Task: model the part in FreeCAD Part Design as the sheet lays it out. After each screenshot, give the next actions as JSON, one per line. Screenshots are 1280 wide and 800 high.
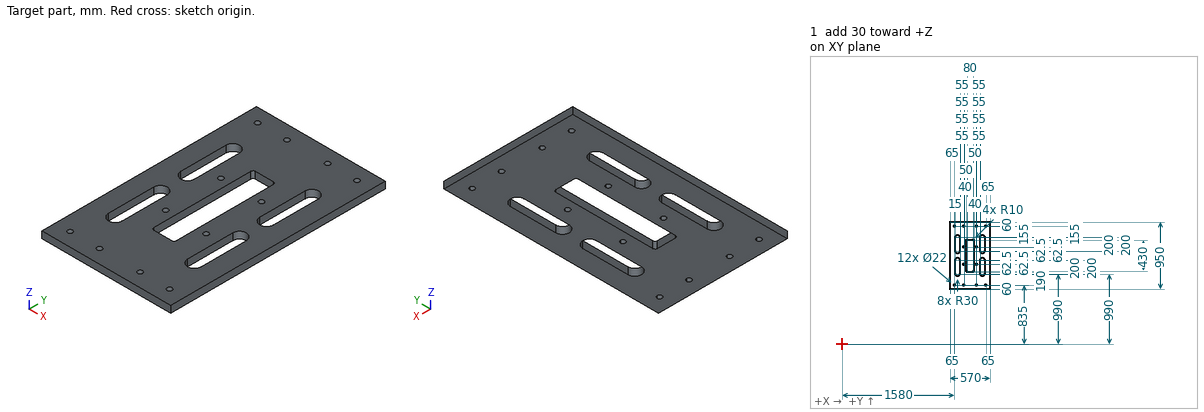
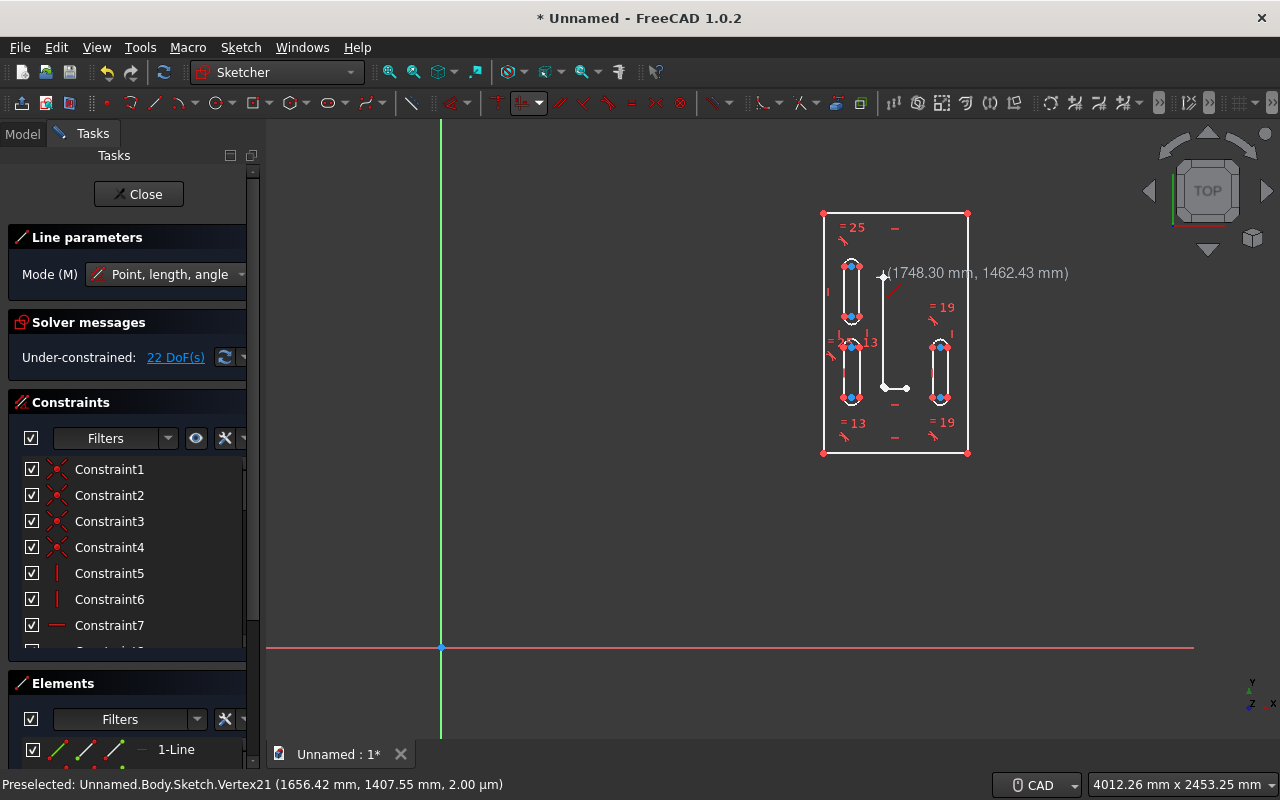
{"action": "scroll", "coordinate": [886, 275], "scroll_direction": "up", "scroll_amount": 8}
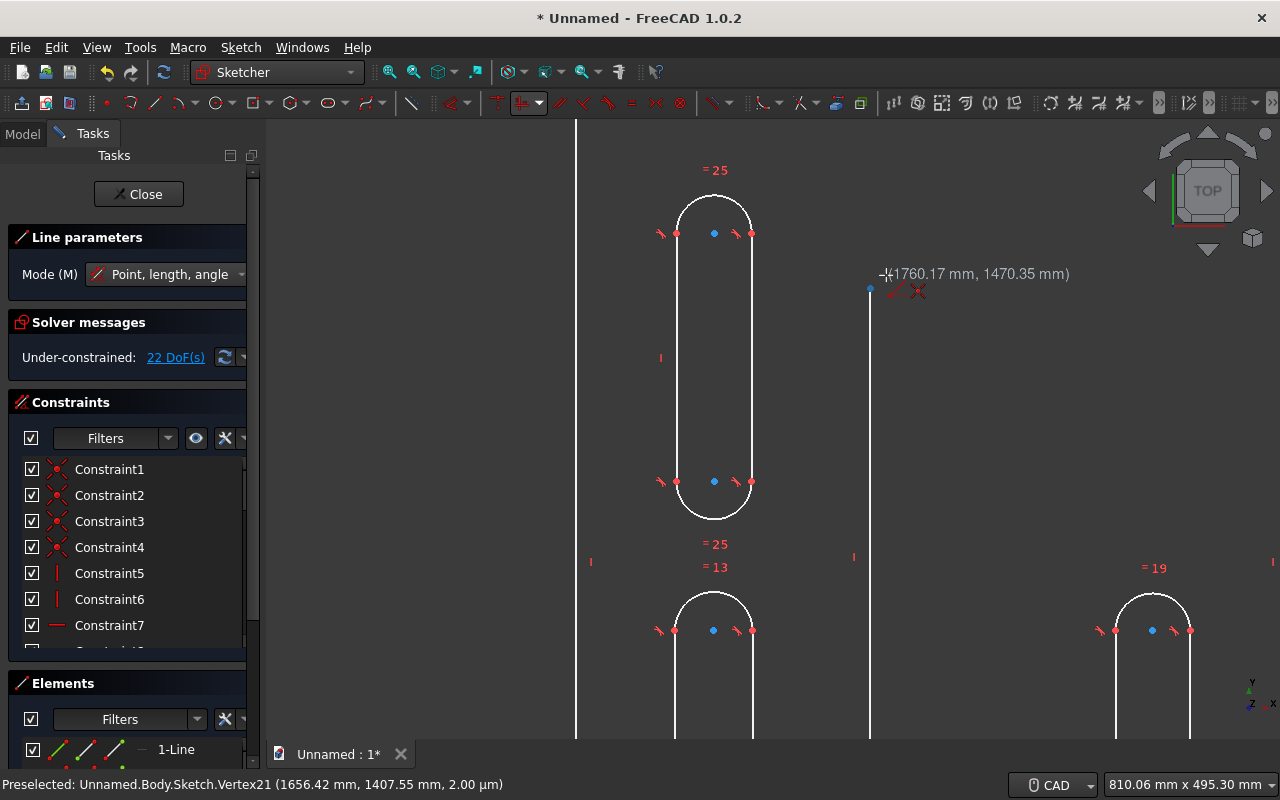
{"action": "left_click", "coordinate": [883, 273]}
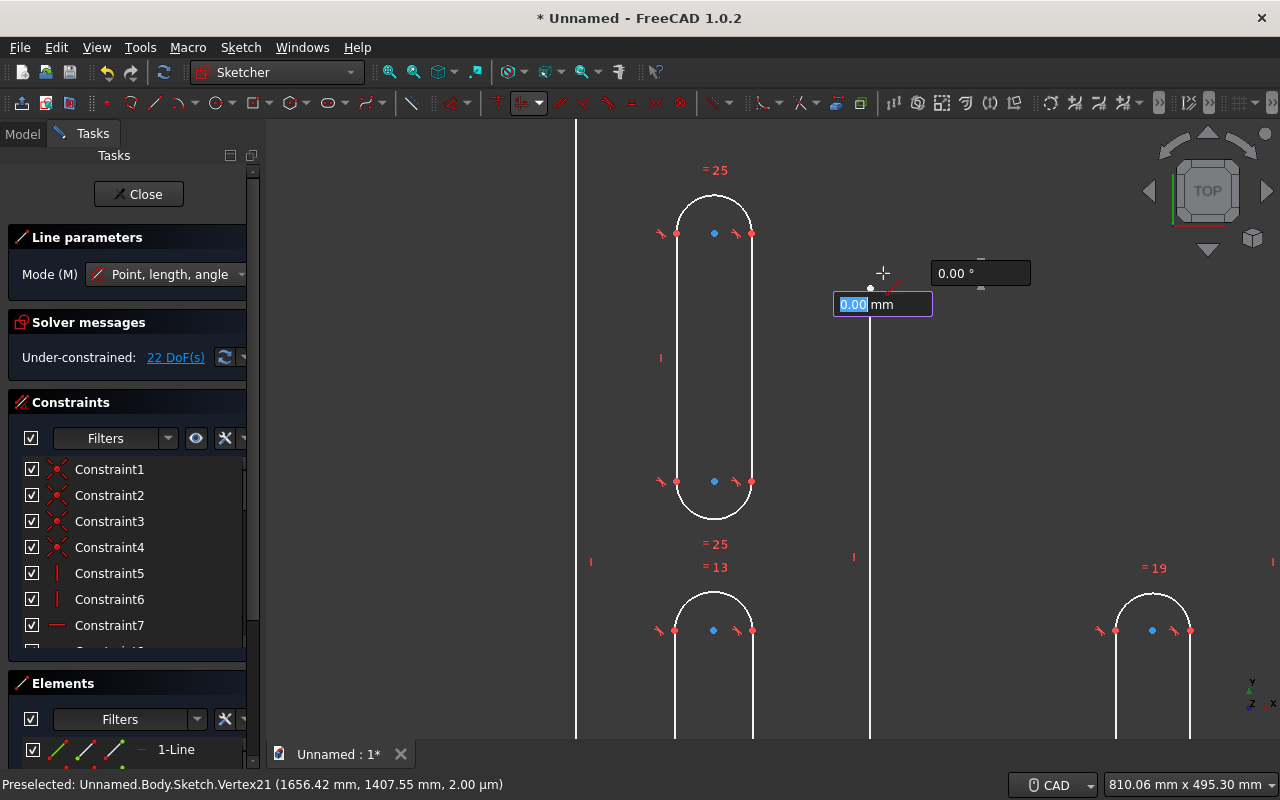
{"action": "scroll", "coordinate": [886, 274], "scroll_direction": "down", "scroll_amount": 8}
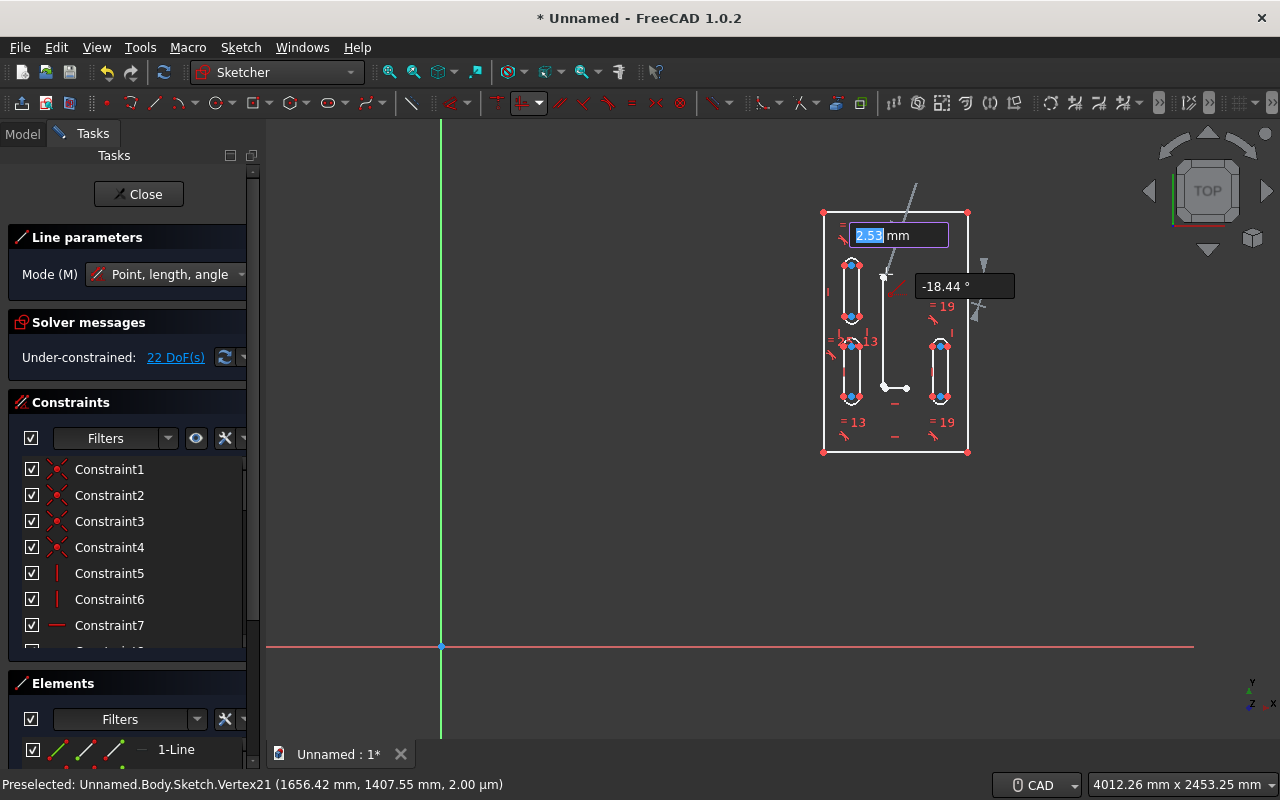
{"action": "left_click", "coordinate": [906, 274]}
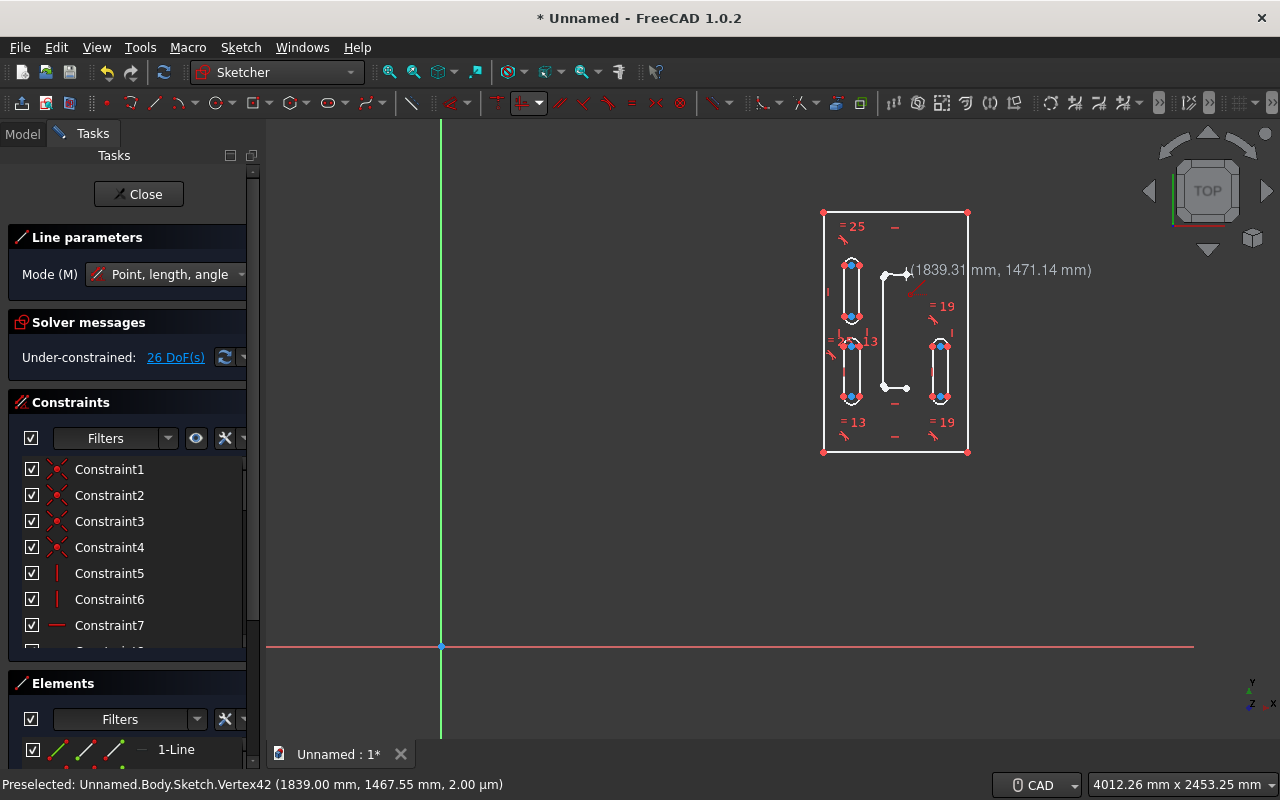
{"action": "scroll", "coordinate": [909, 277], "scroll_direction": "up", "scroll_amount": 8}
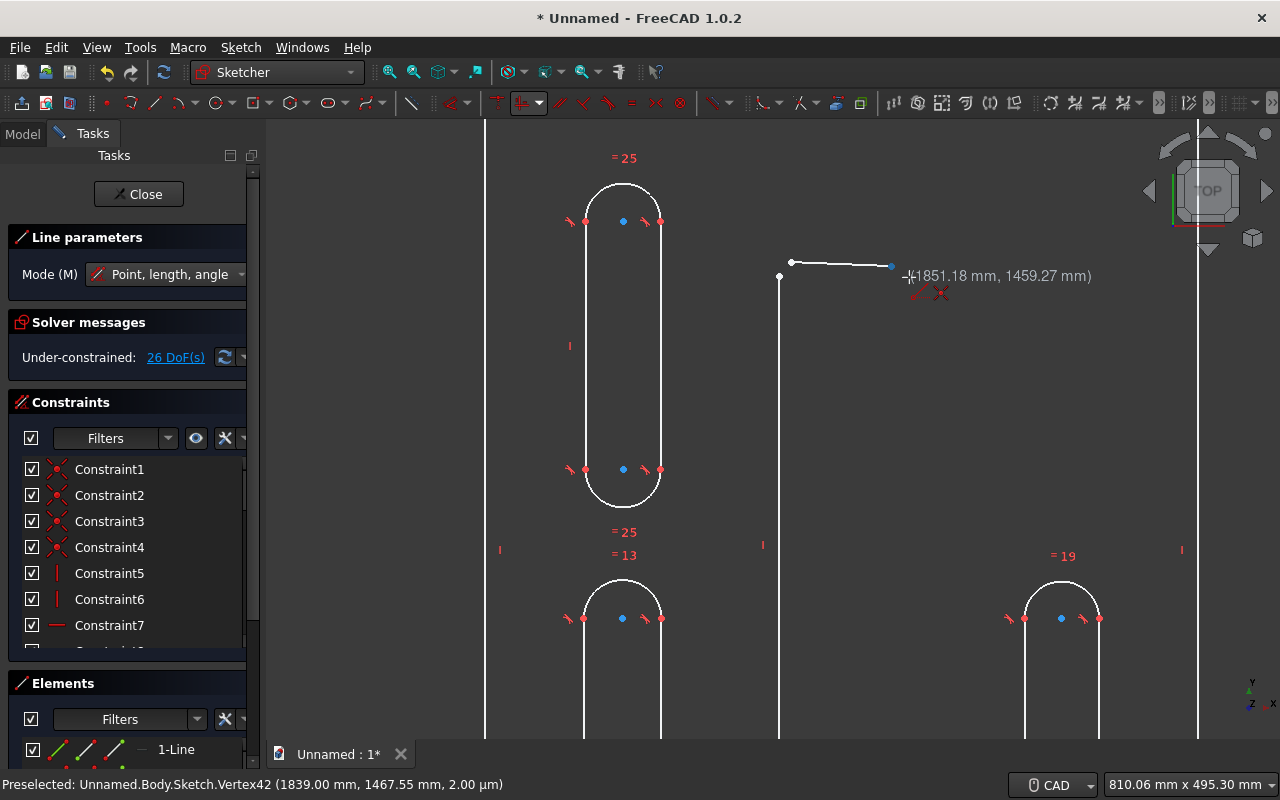
{"action": "left_click", "coordinate": [905, 274]}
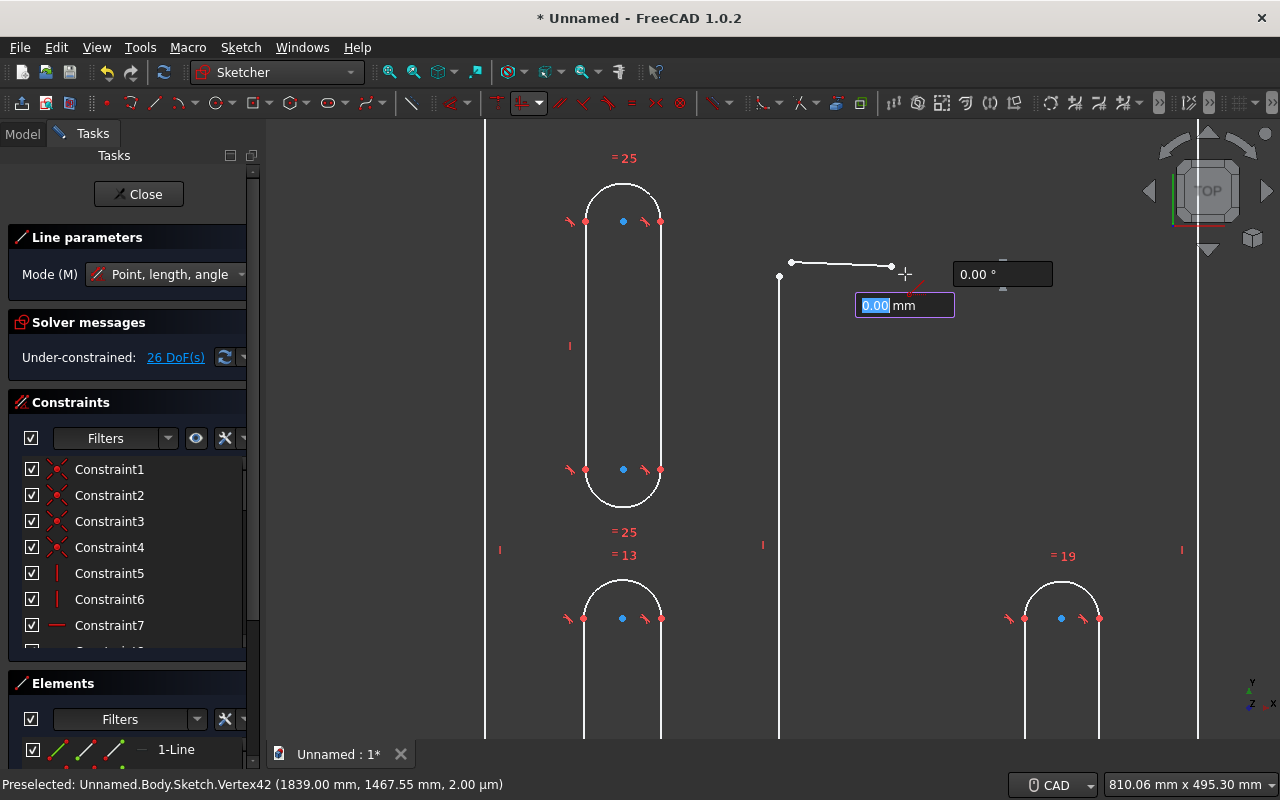
{"action": "scroll", "coordinate": [909, 277], "scroll_direction": "down", "scroll_amount": 8}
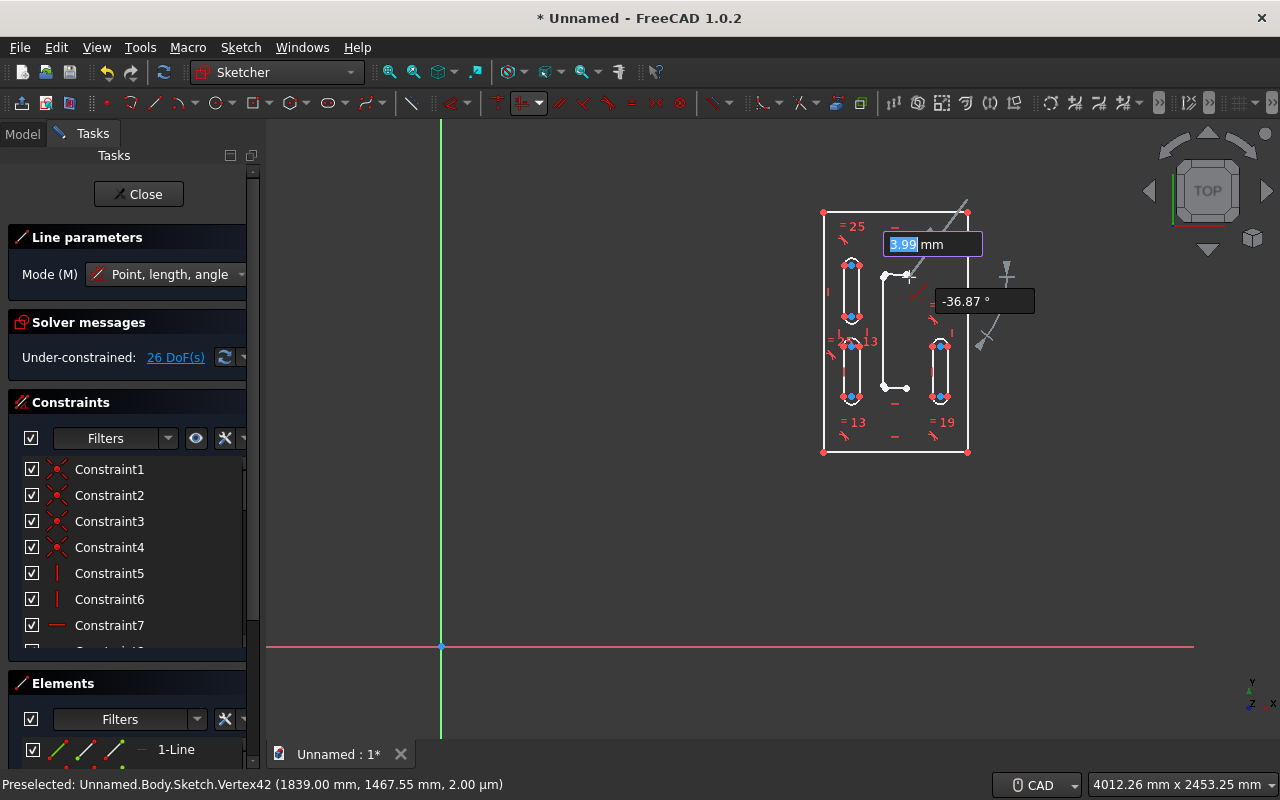
{"action": "scroll", "coordinate": [909, 385], "scroll_direction": "up", "scroll_amount": 8}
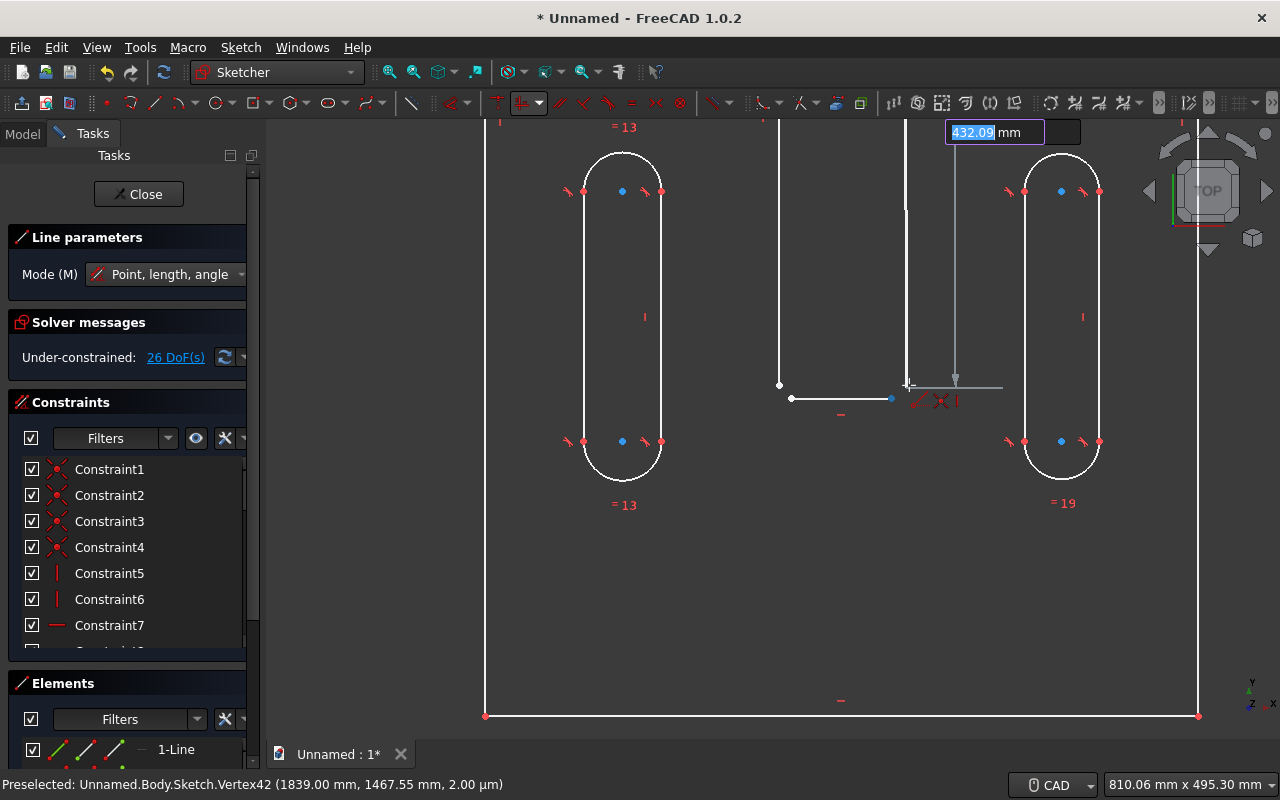
{"action": "left_click", "coordinate": [905, 384]}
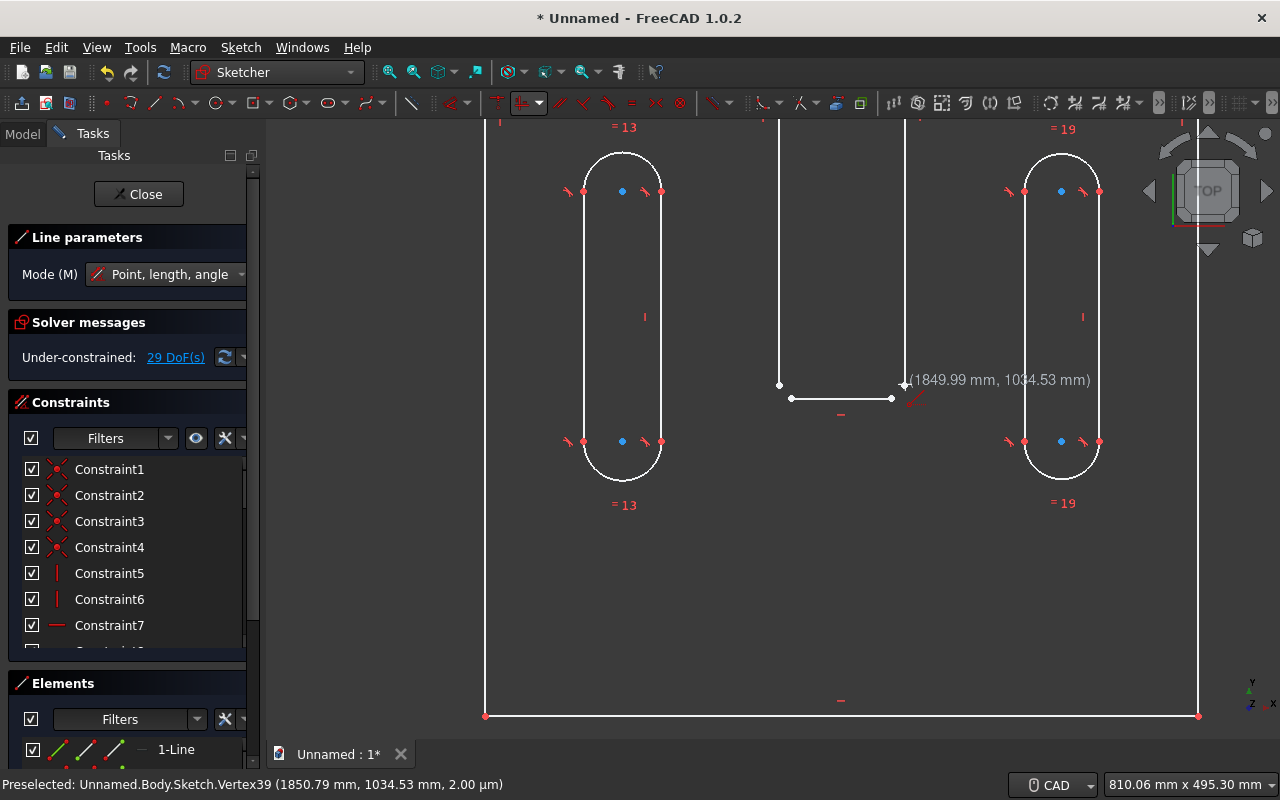
{"action": "left_click", "coordinate": [198, 104]}